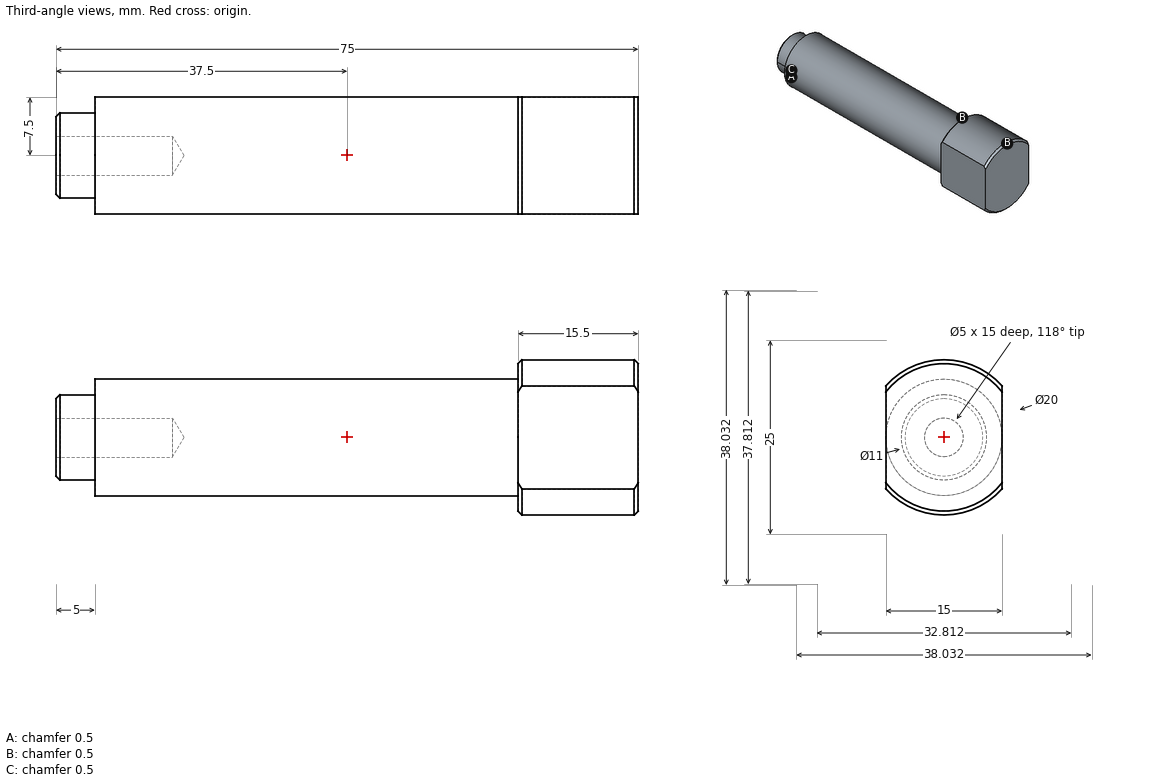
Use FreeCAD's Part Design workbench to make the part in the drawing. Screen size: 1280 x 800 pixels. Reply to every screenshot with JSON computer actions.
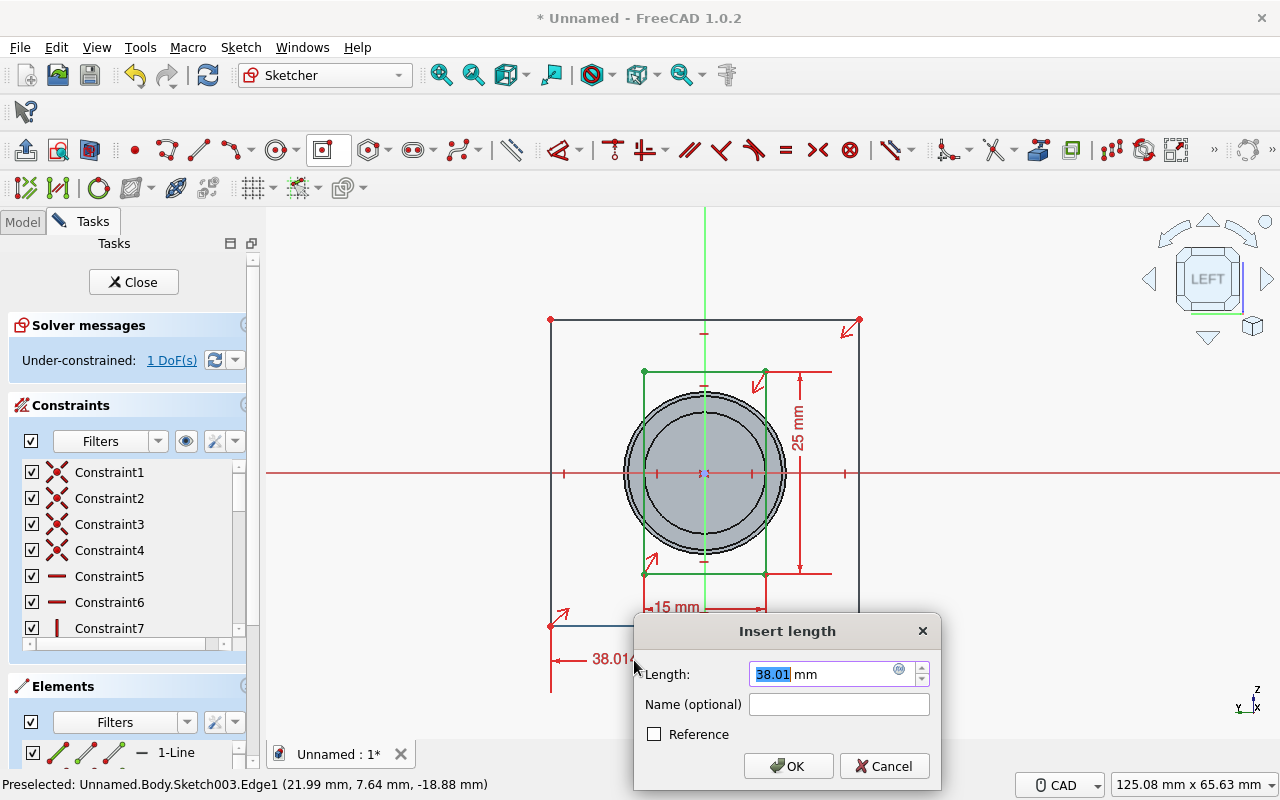
{"action": "type", "text": "38.032"}
{"action": "key", "text": "Return"}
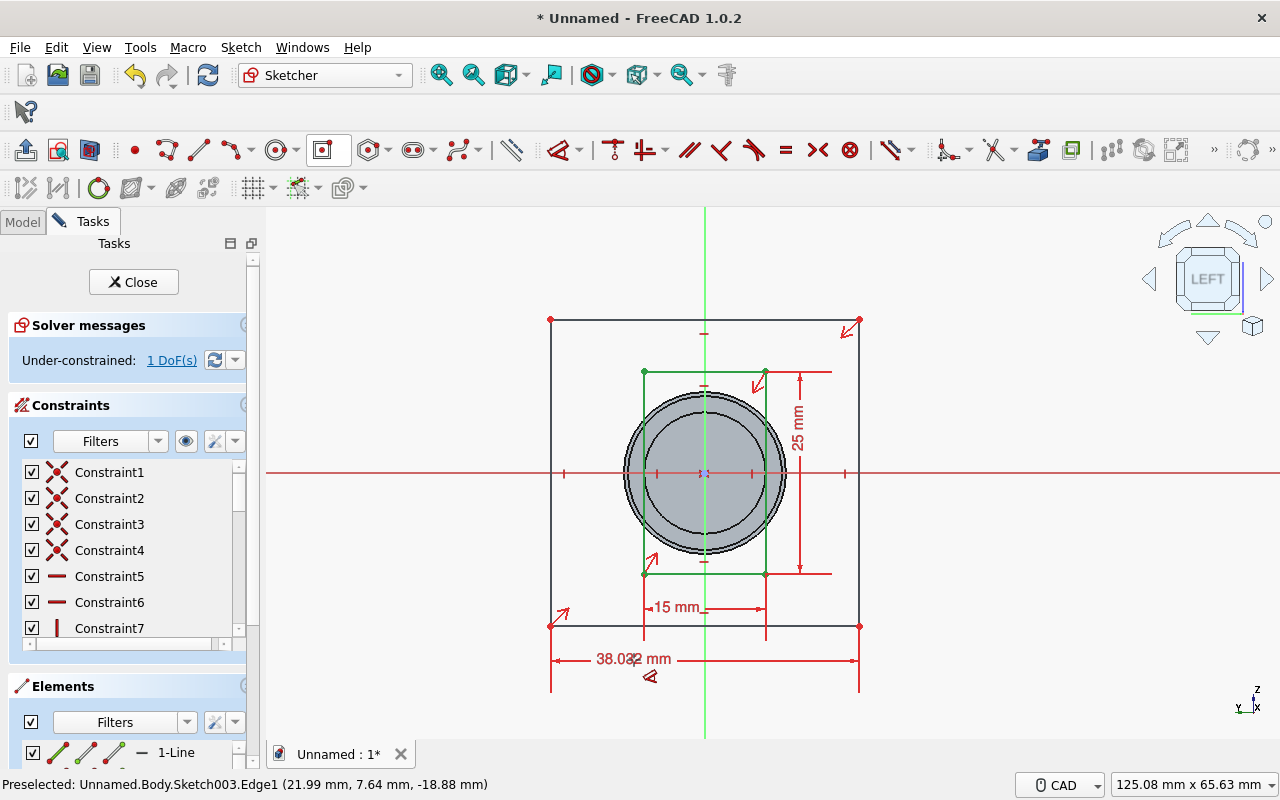
{"action": "left_click", "coordinate": [859, 534]}
{"action": "left_click", "coordinate": [893, 403]}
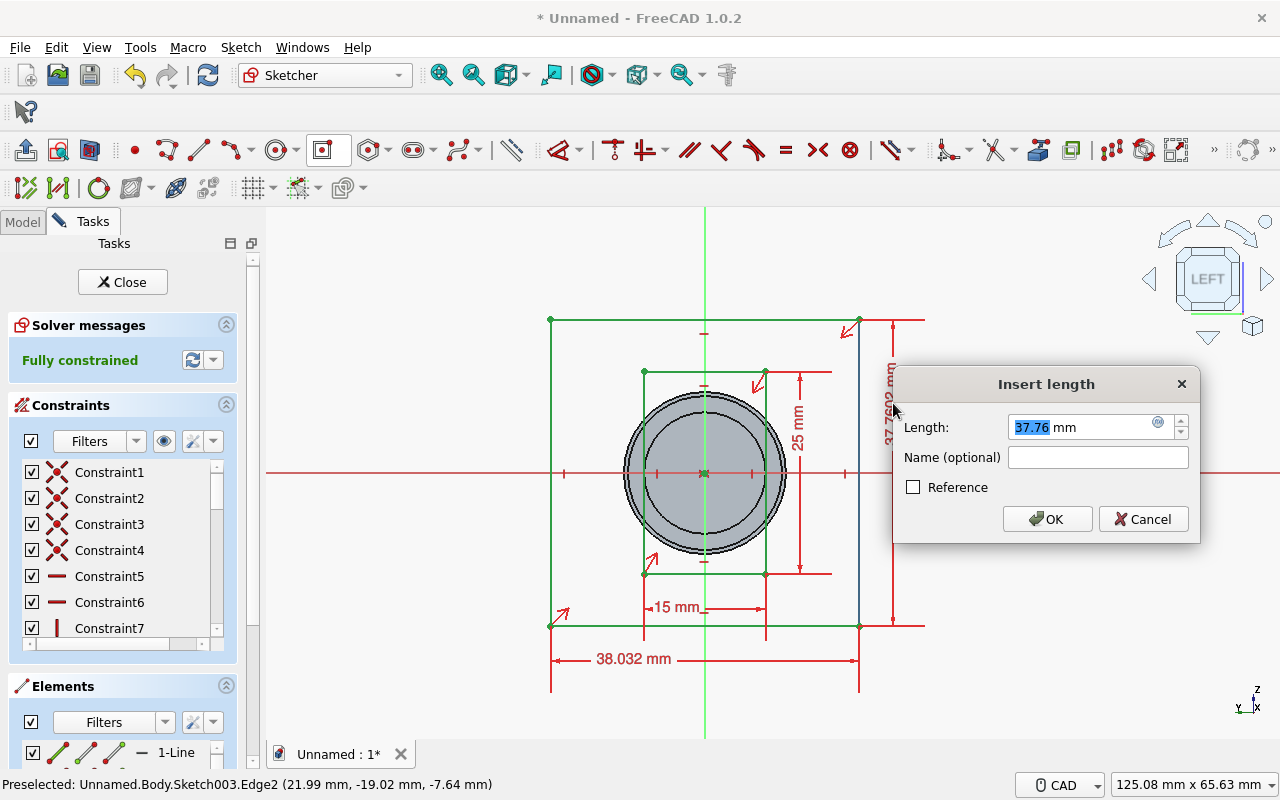
{"action": "type", "text": "38.032"}
{"action": "key", "text": "Return"}
{"action": "key", "text": "Escape"}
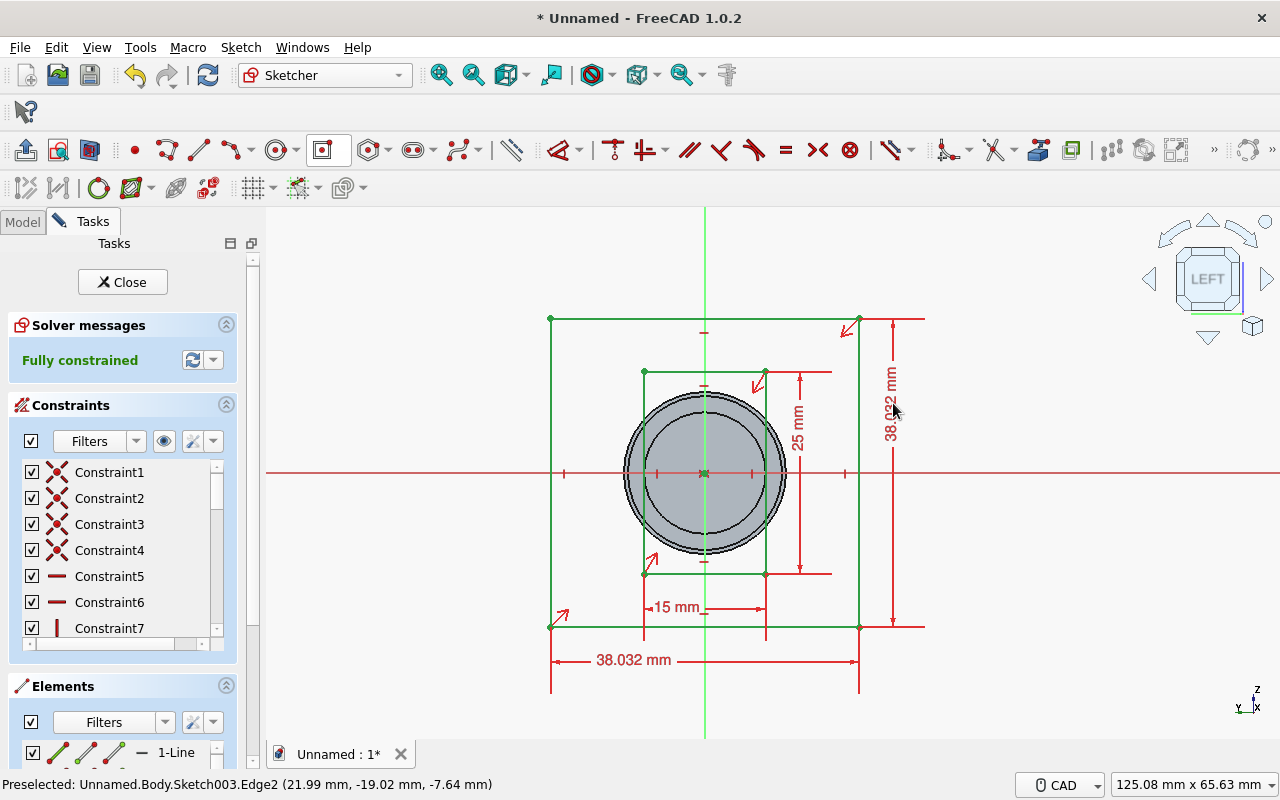
{"action": "left_click", "coordinate": [123, 282]}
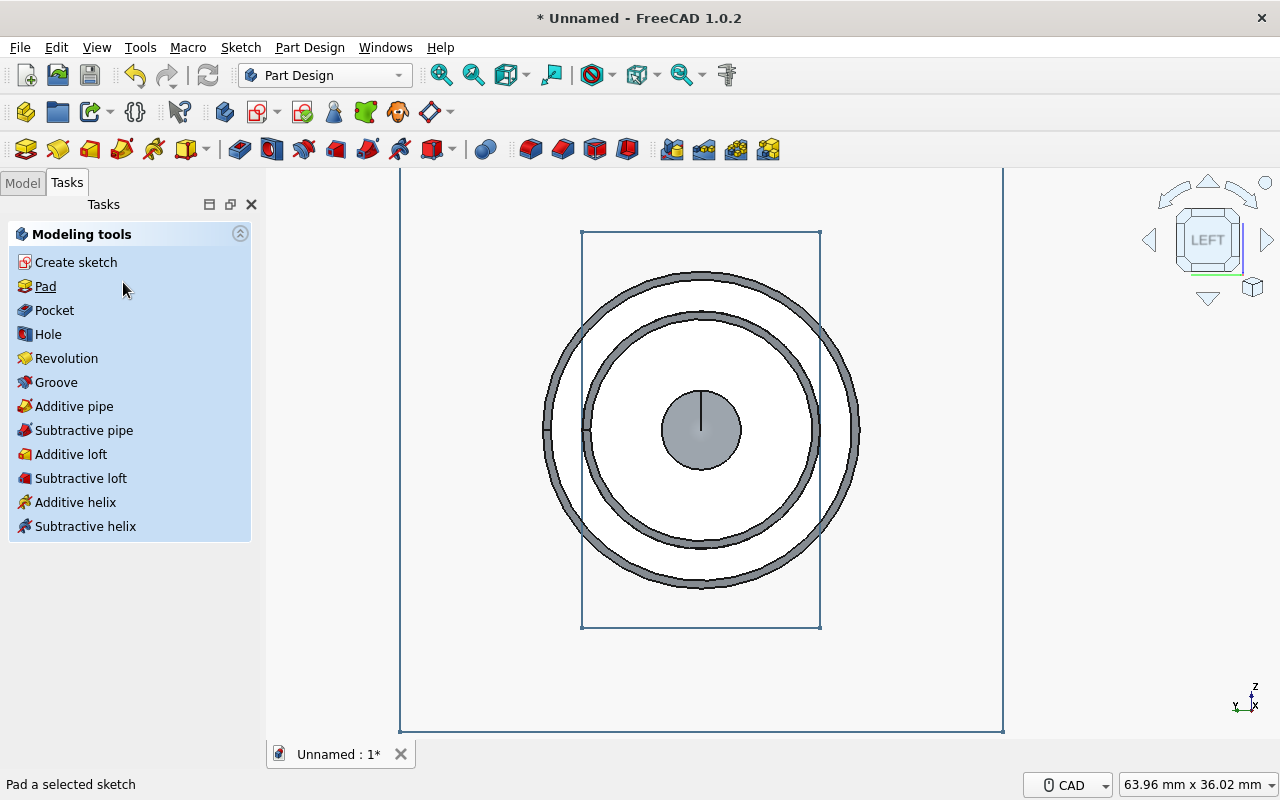
{"action": "left_click", "coordinate": [240, 150]}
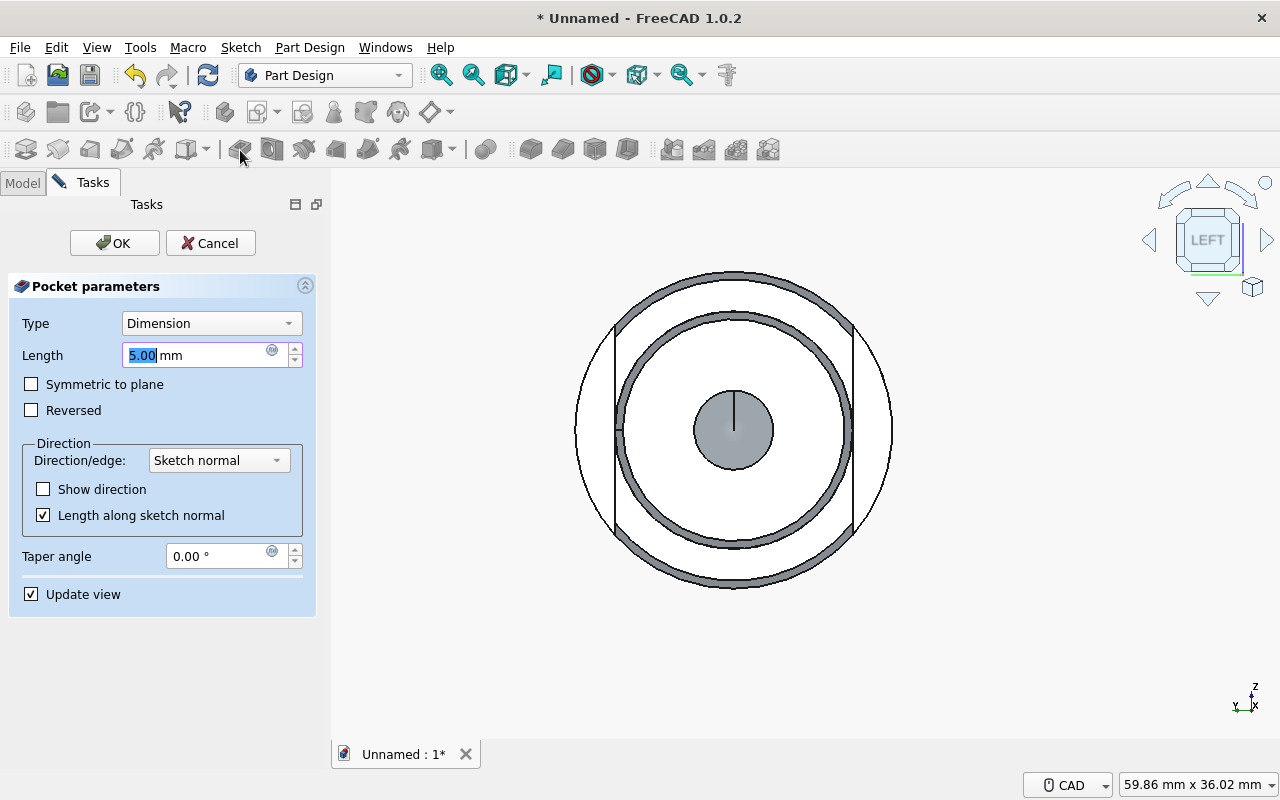
{"action": "left_click", "coordinate": [212, 324]}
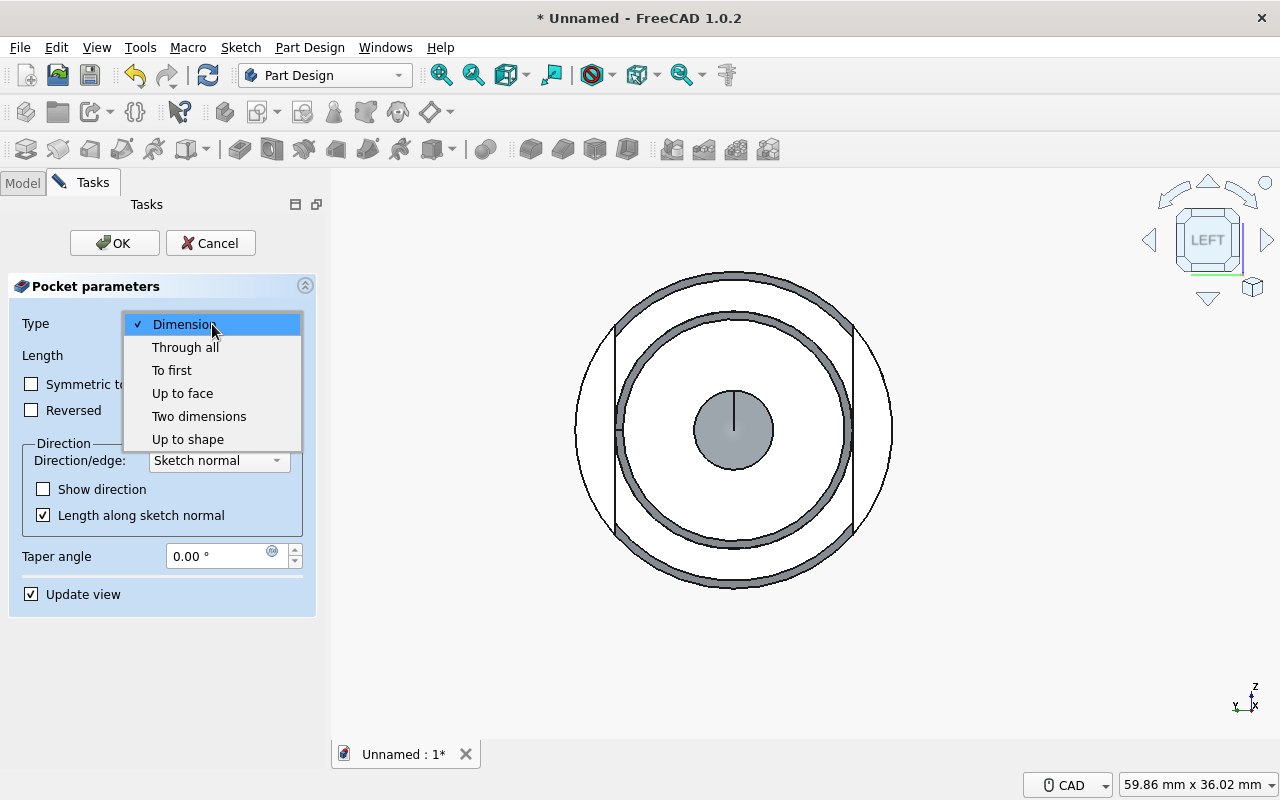
{"action": "left_click", "coordinate": [212, 348]}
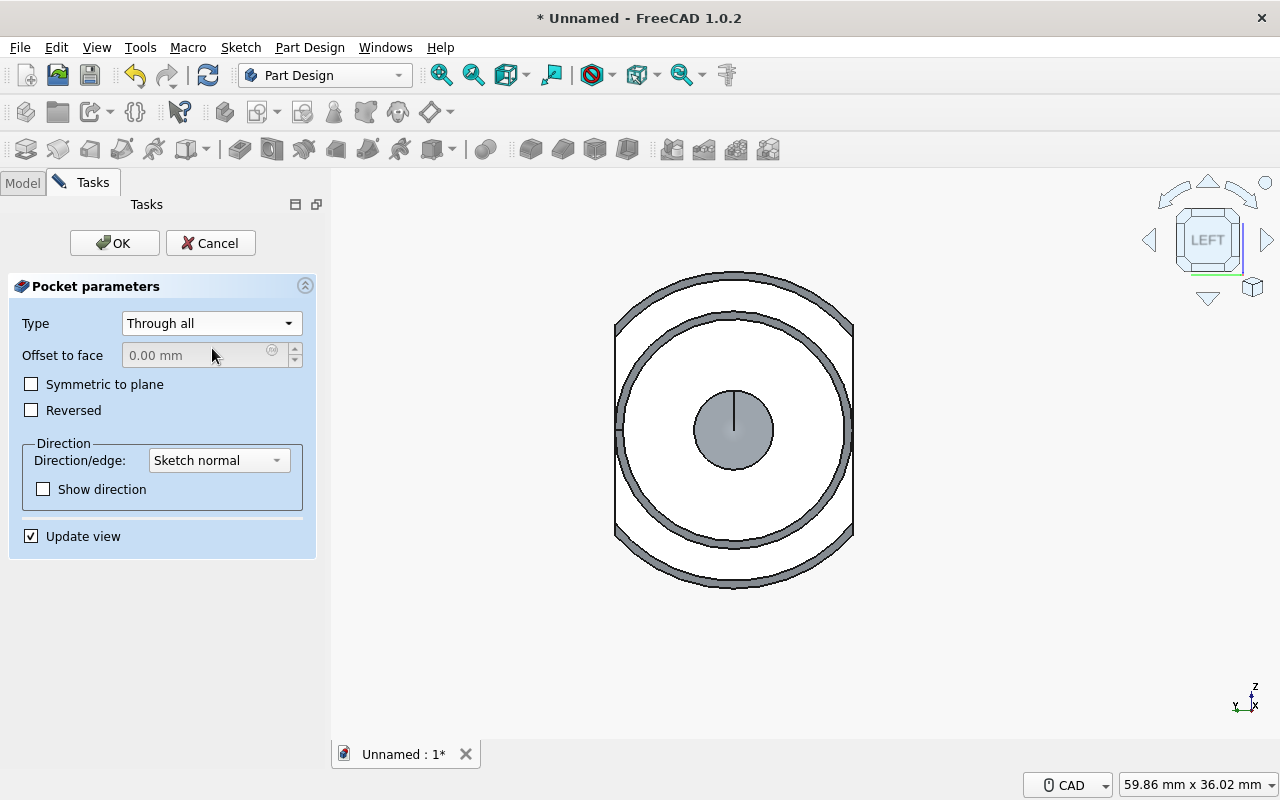
{"action": "left_click", "coordinate": [115, 243]}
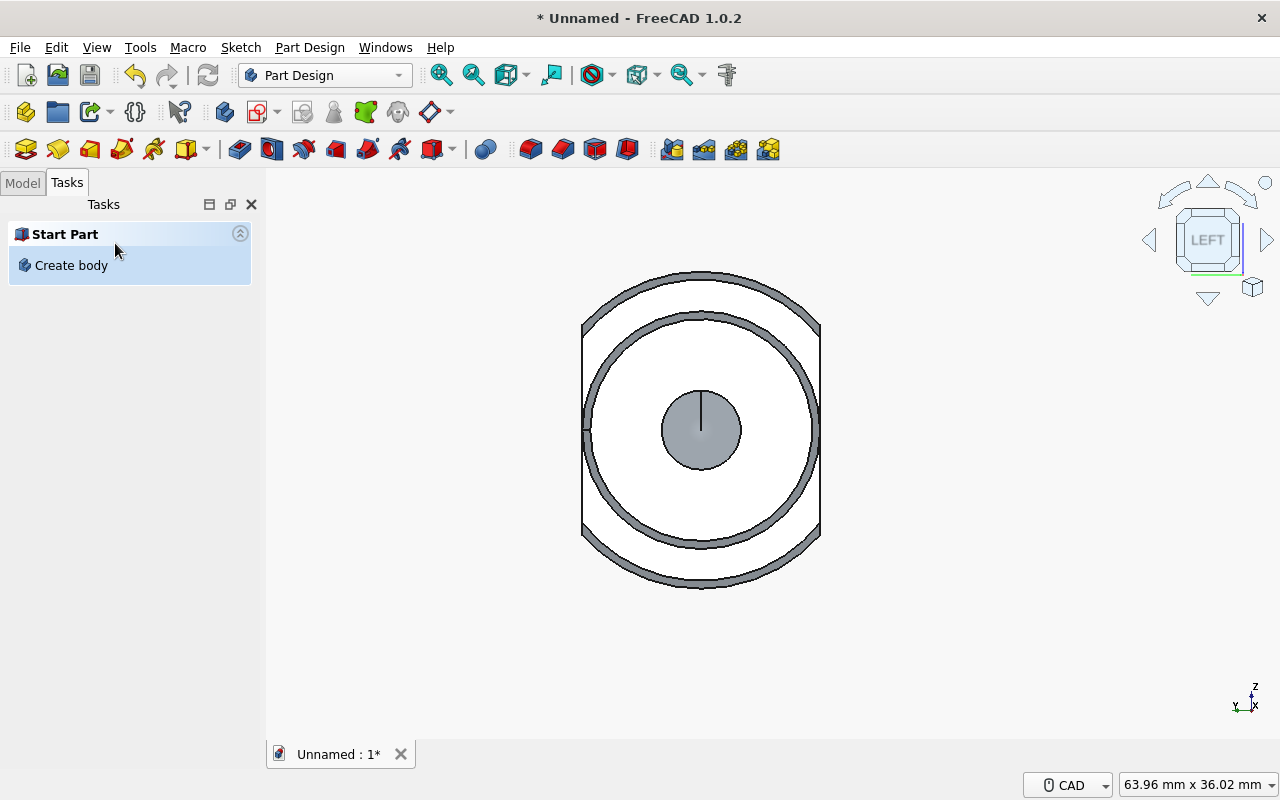
{"action": "left_click", "coordinate": [765, 461]}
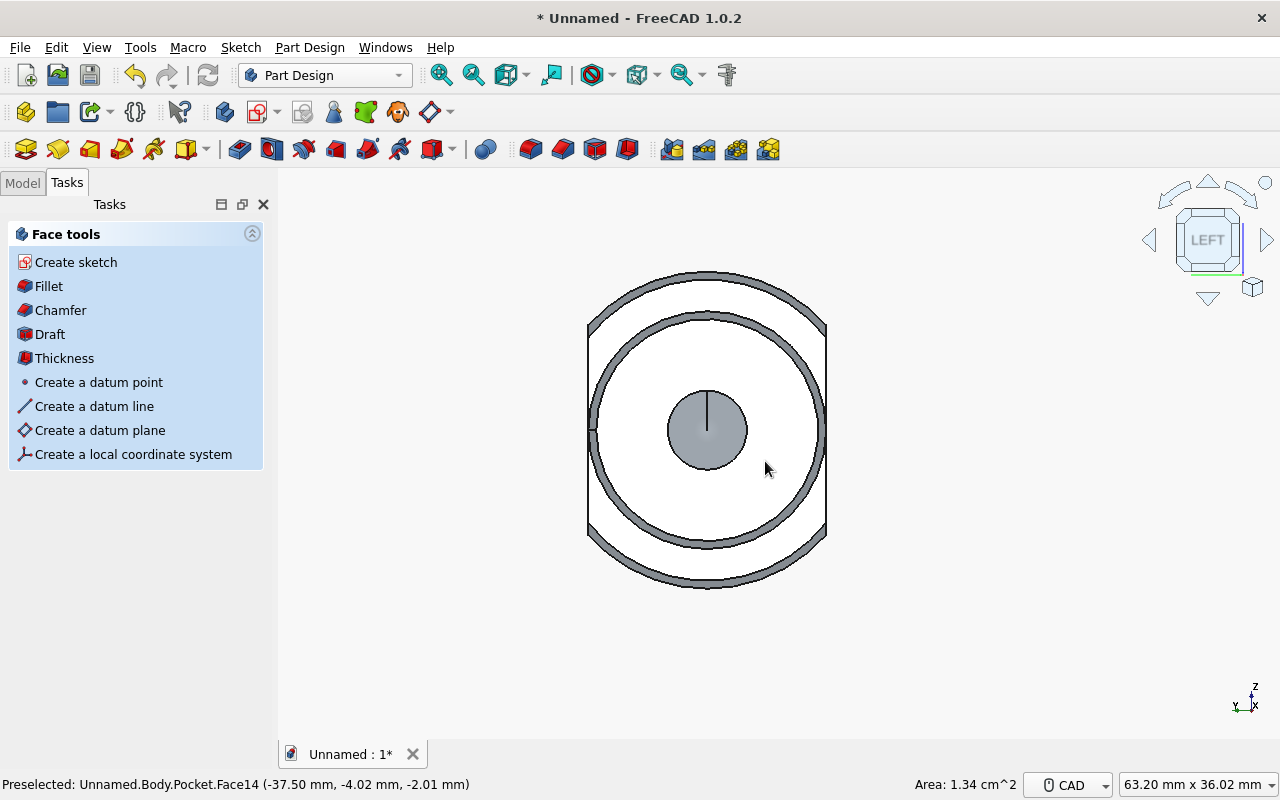
{"action": "left_click", "coordinate": [258, 112]}